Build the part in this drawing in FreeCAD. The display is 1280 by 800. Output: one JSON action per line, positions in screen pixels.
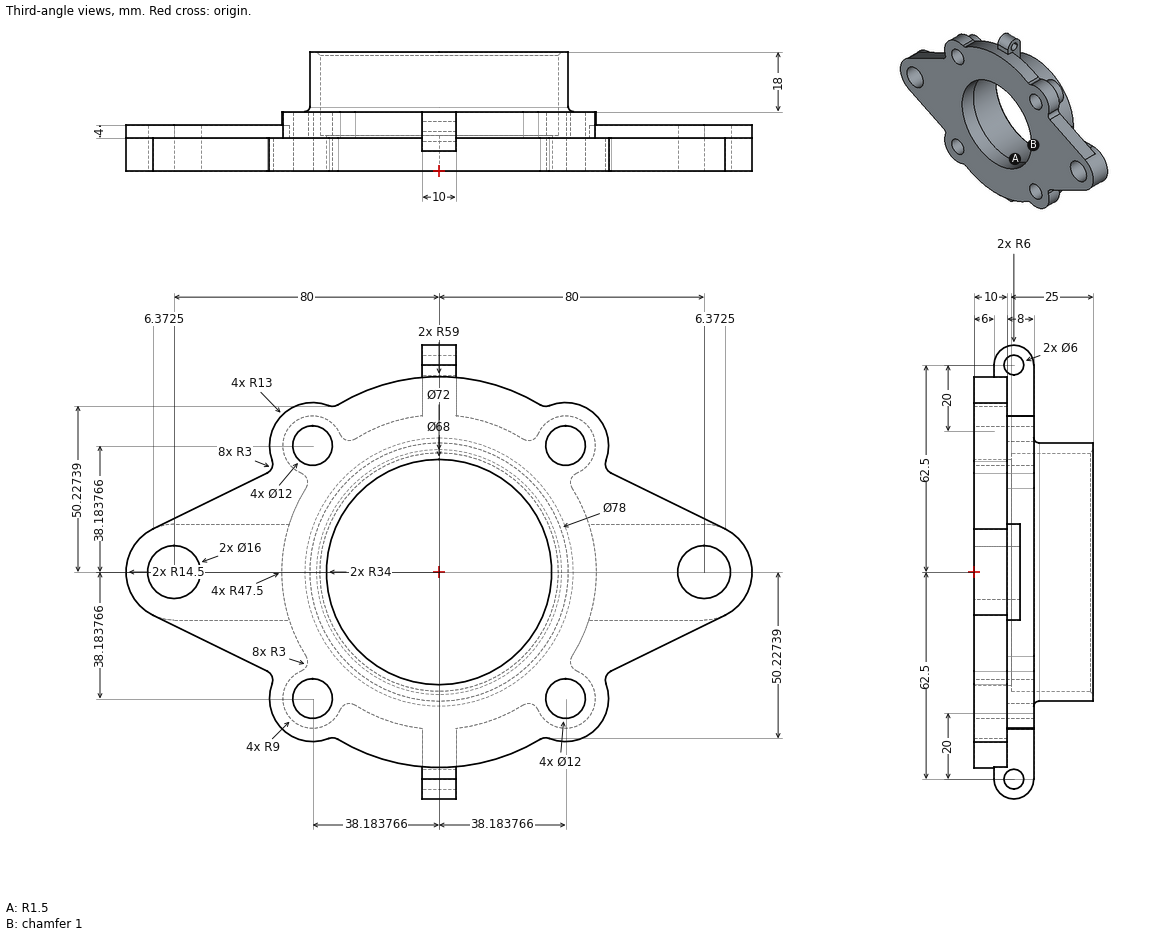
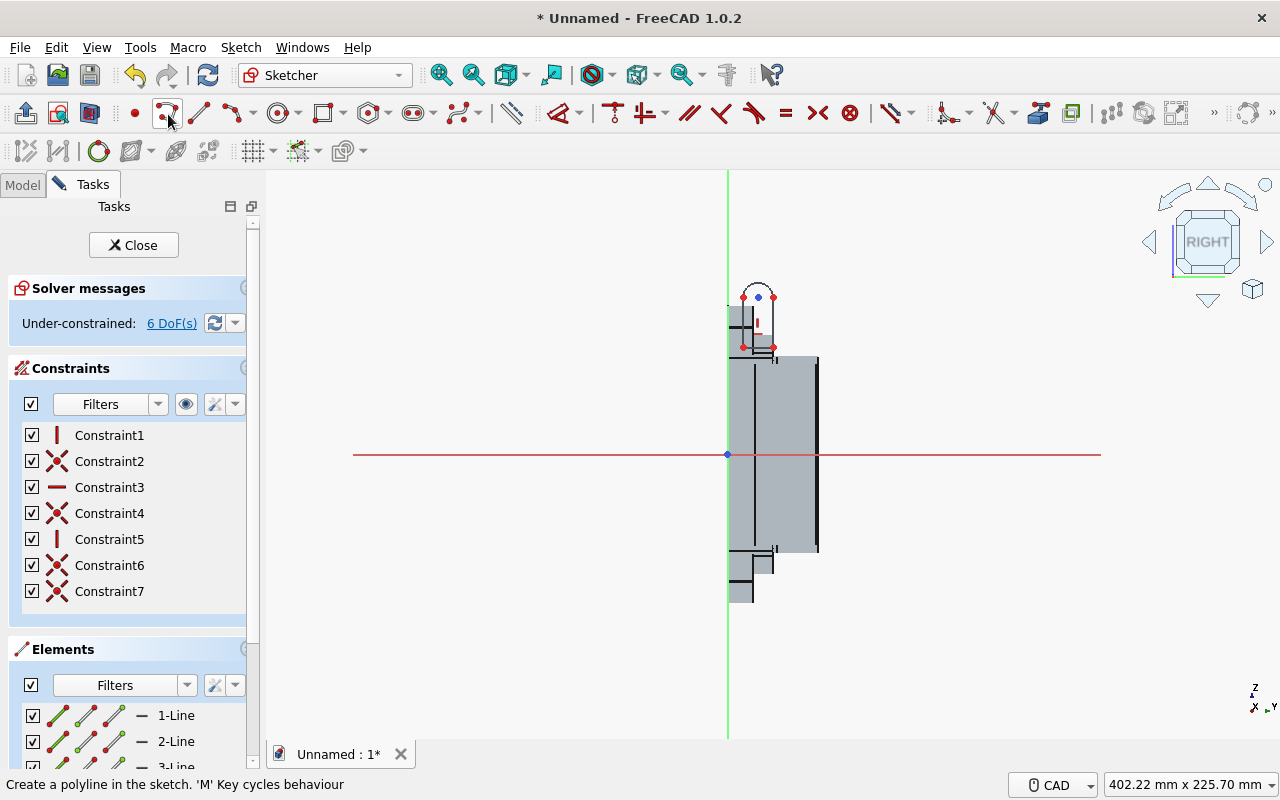
{"action": "left_click", "coordinate": [773, 612]}
{"action": "left_click", "coordinate": [773, 562]}
{"action": "left_click", "coordinate": [743, 562]}
{"action": "left_click", "coordinate": [743, 612]}
{"action": "right_click", "coordinate": [743, 612]}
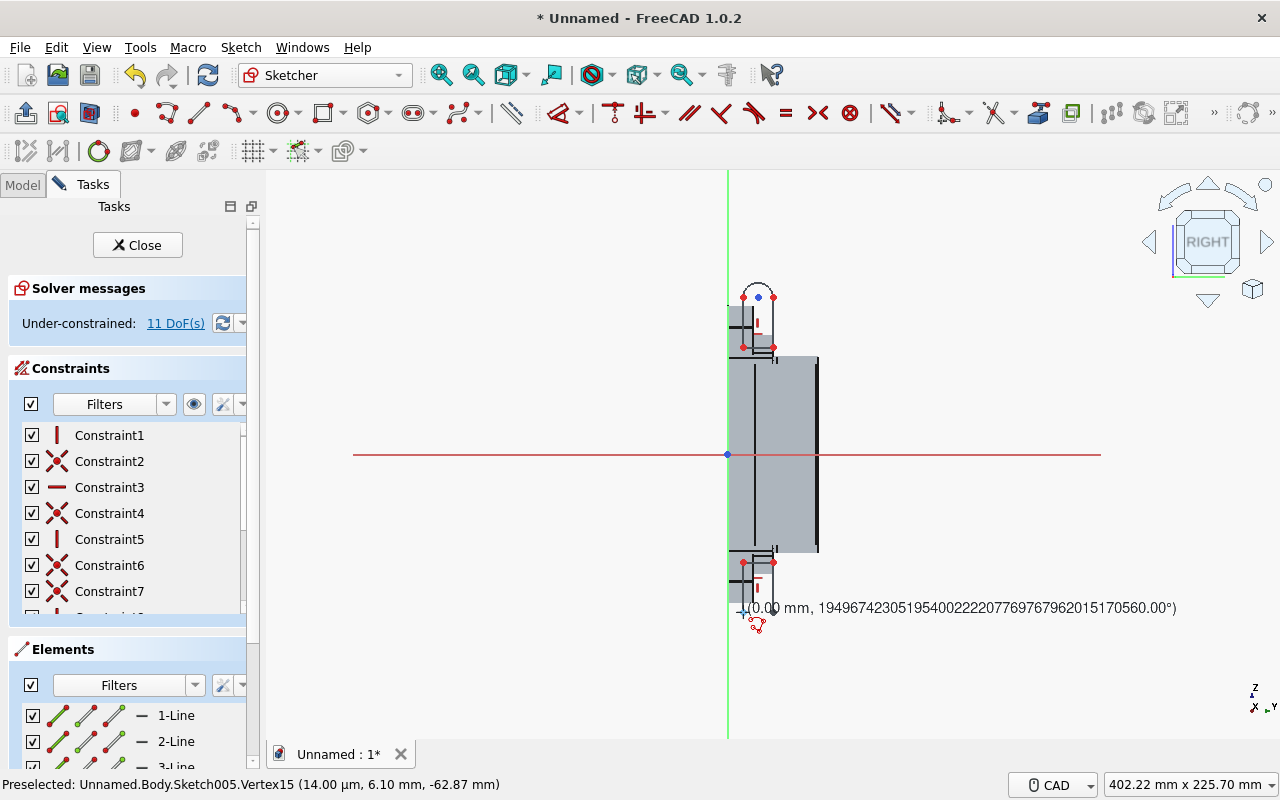
{"action": "left_click", "coordinate": [232, 114]}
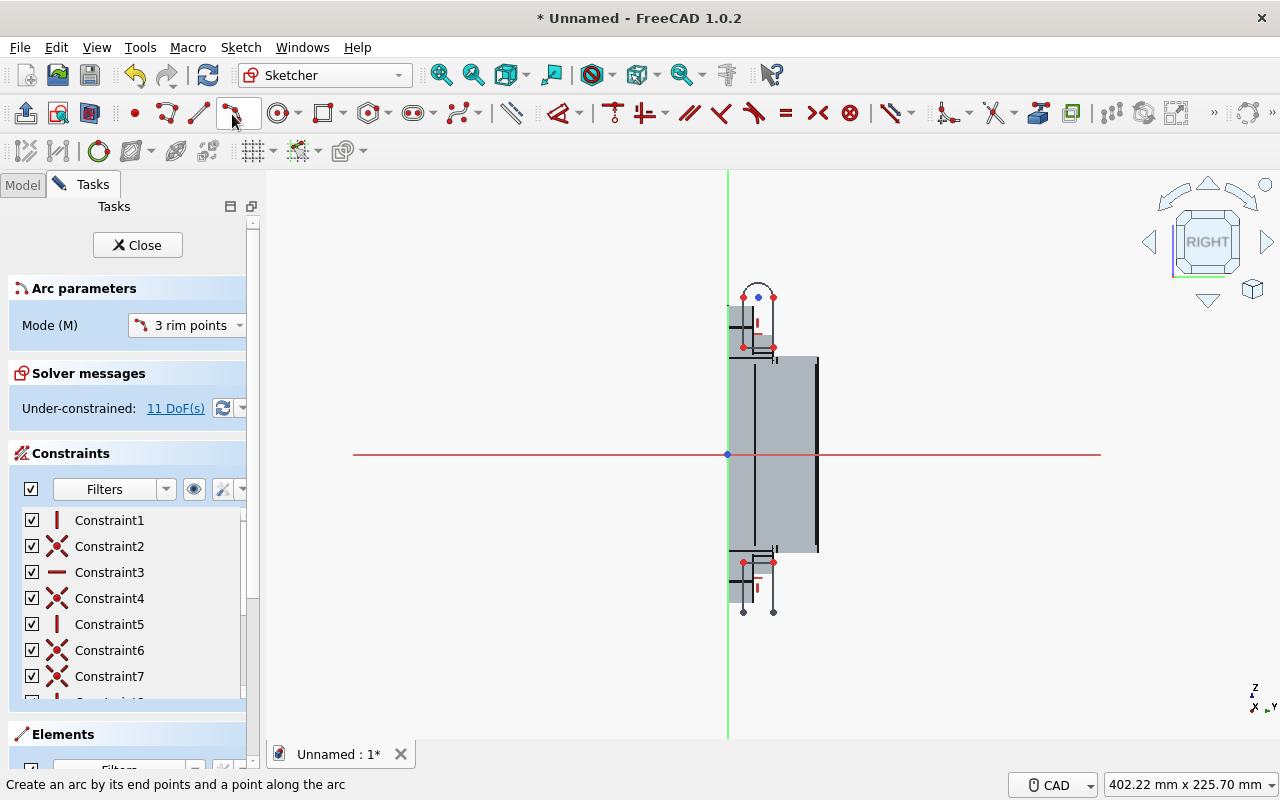
{"action": "left_click", "coordinate": [743, 613]}
{"action": "left_click", "coordinate": [773, 613]}
{"action": "left_click", "coordinate": [758, 627]}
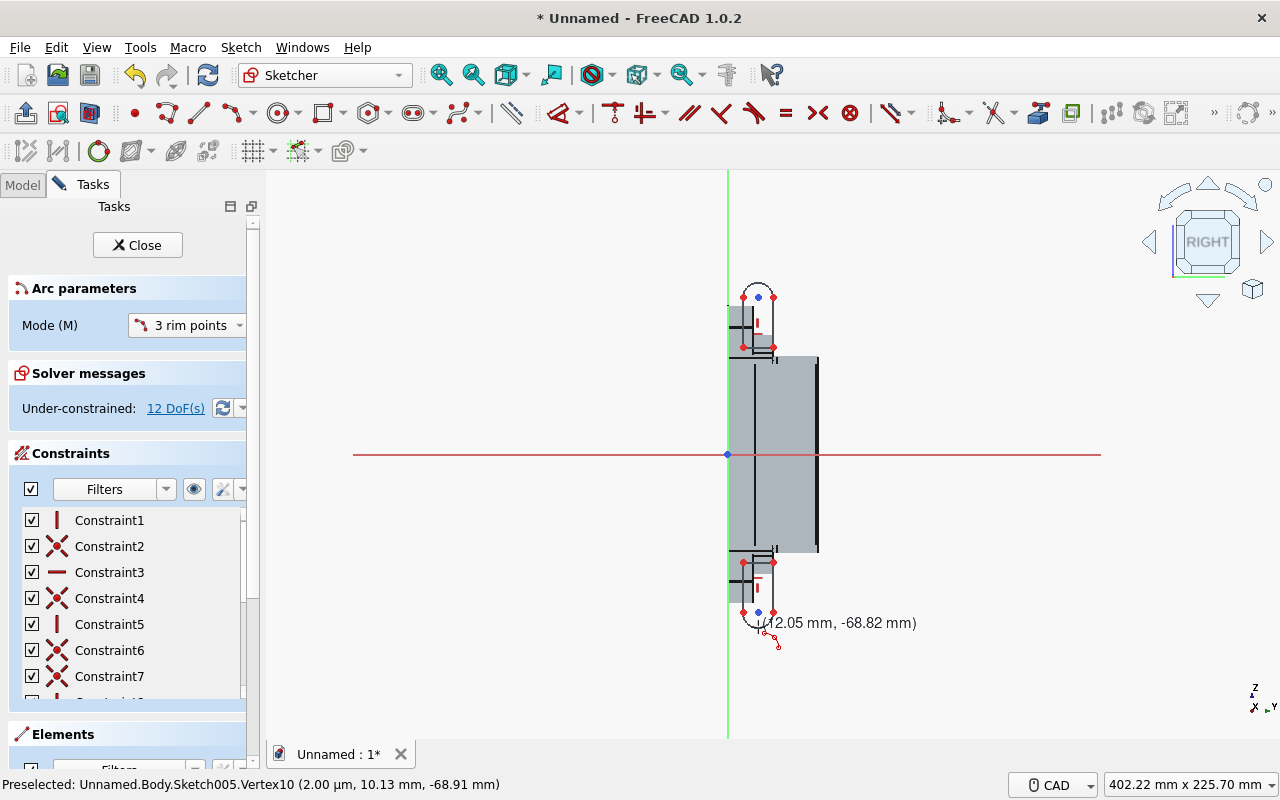
{"action": "left_click", "coordinate": [278, 114]}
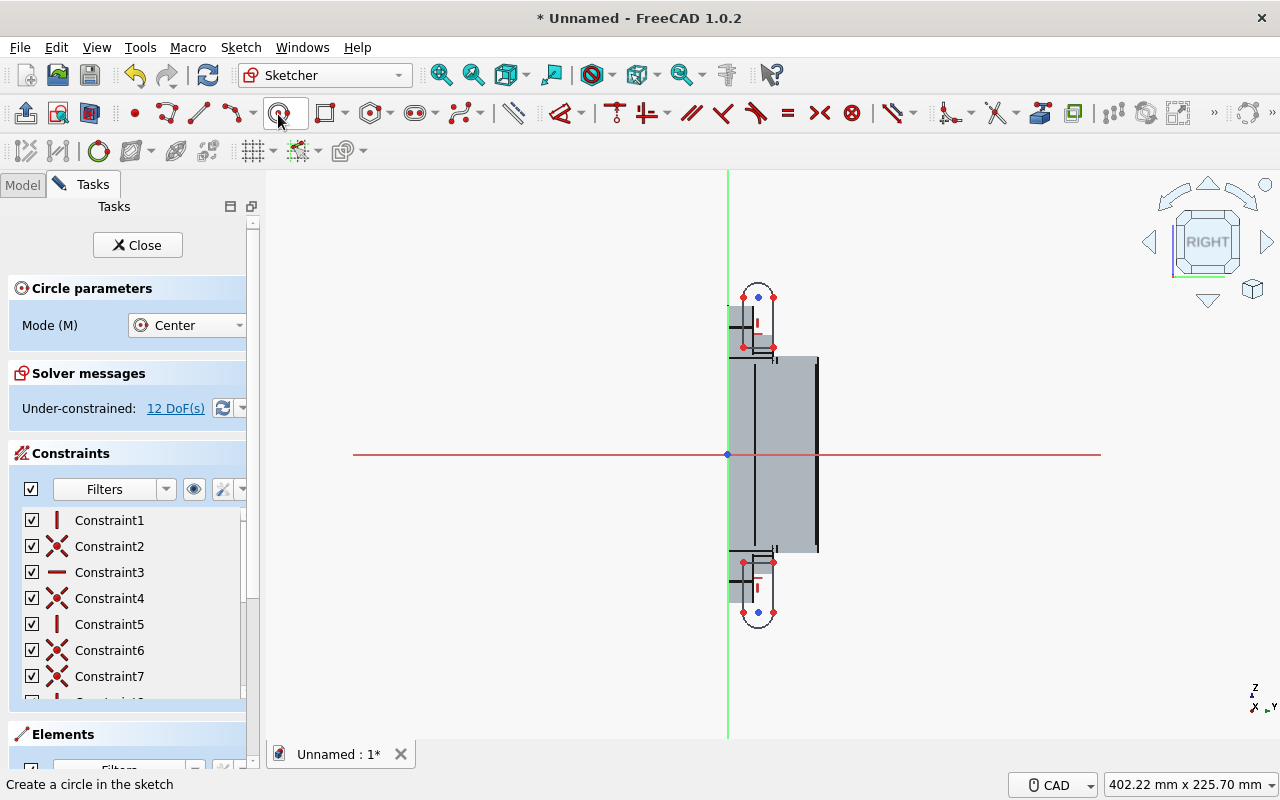
{"action": "scroll", "coordinate": [758, 297], "scroll_direction": "up", "scroll_amount": 6}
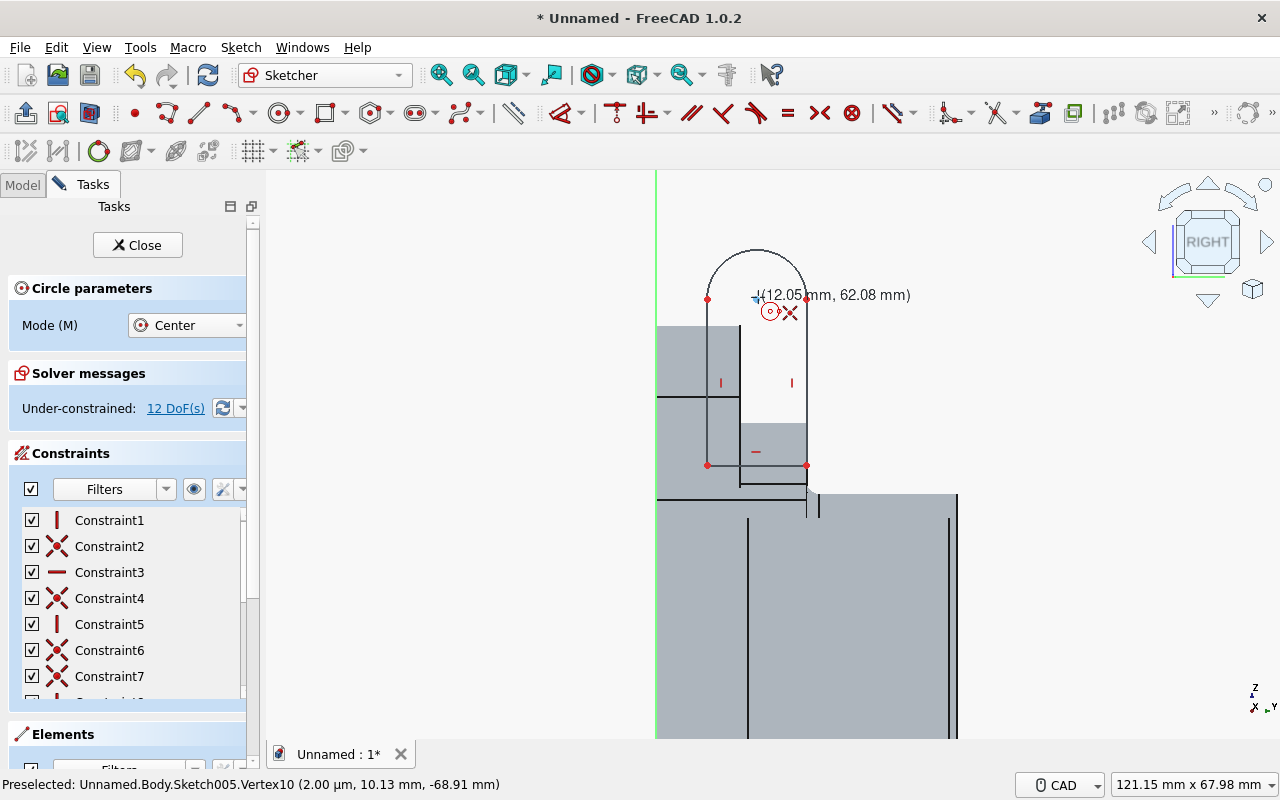
{"action": "left_click", "coordinate": [756, 296]}
{"action": "mouse_move", "coordinate": [774, 279]}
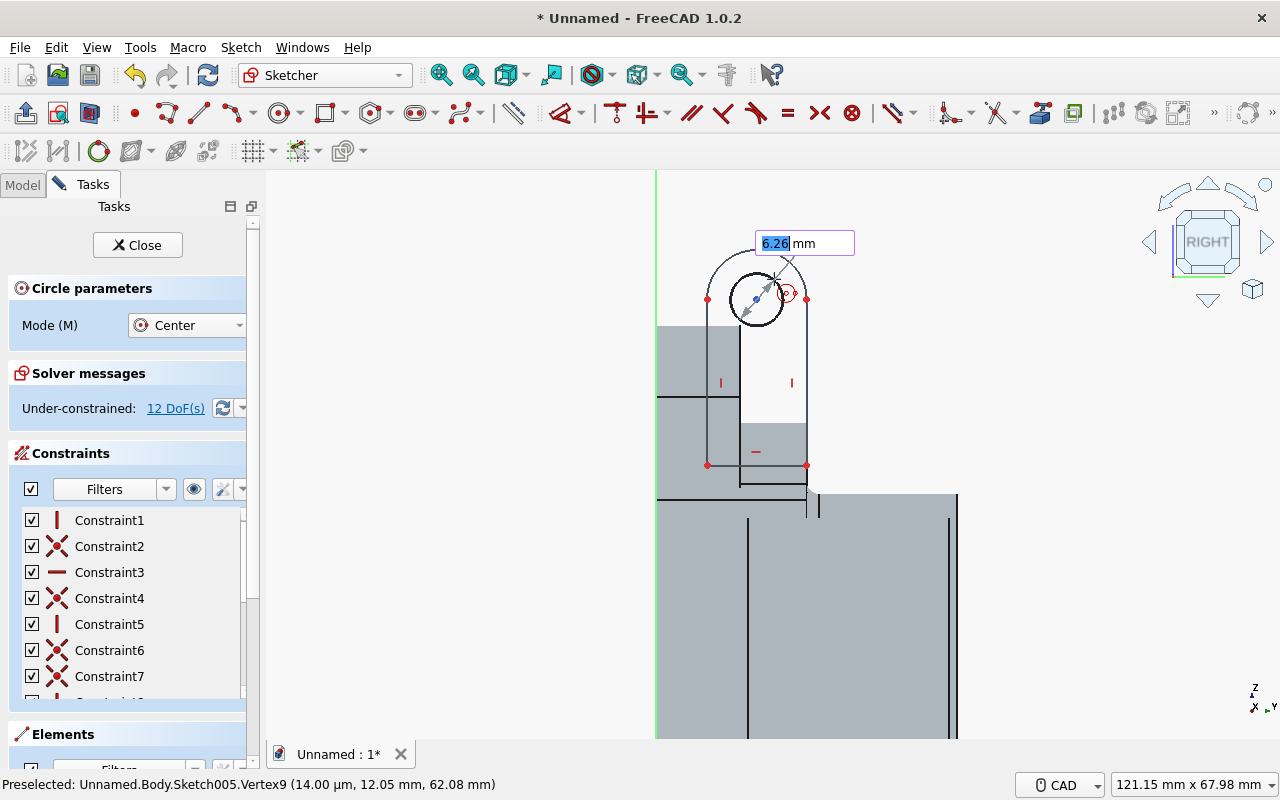
{"action": "type", "text": "6"}
{"action": "key", "text": "Return"}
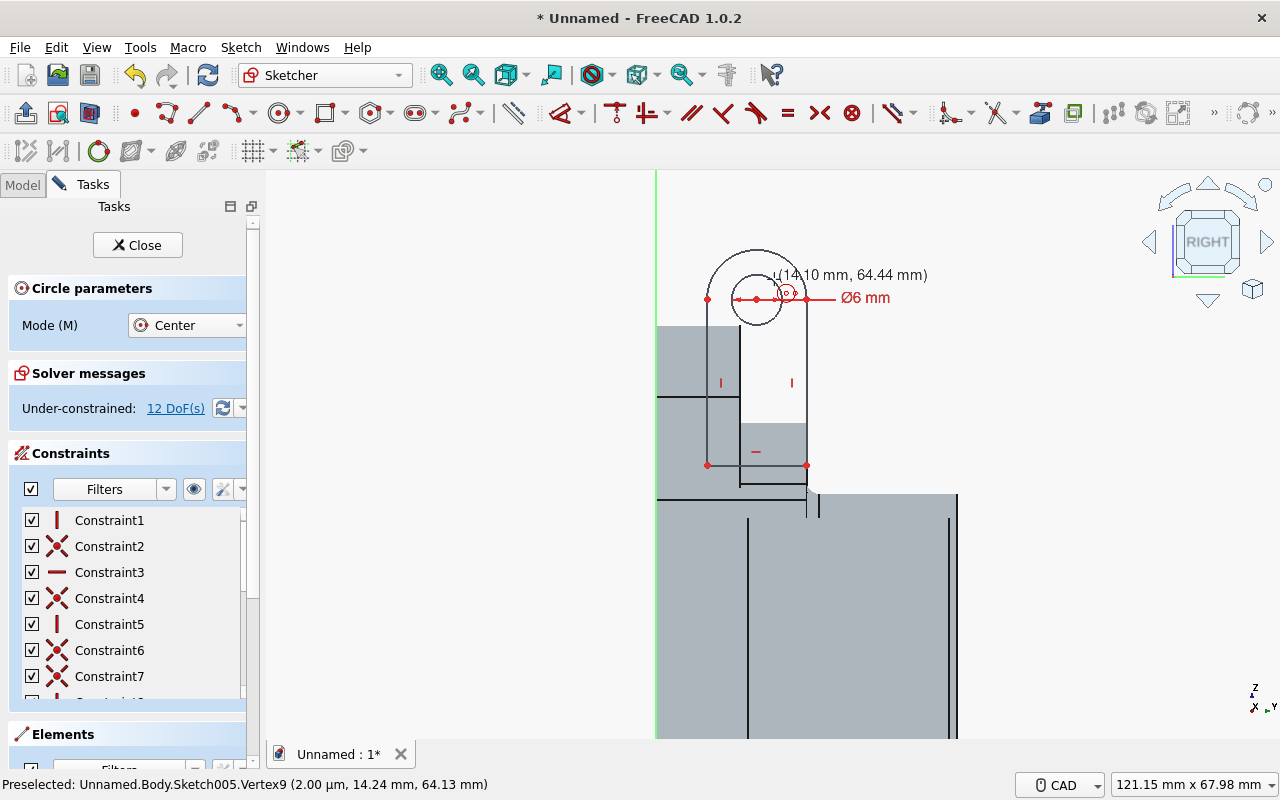
{"action": "scroll", "coordinate": [693, 297], "scroll_direction": "down", "scroll_amount": 6}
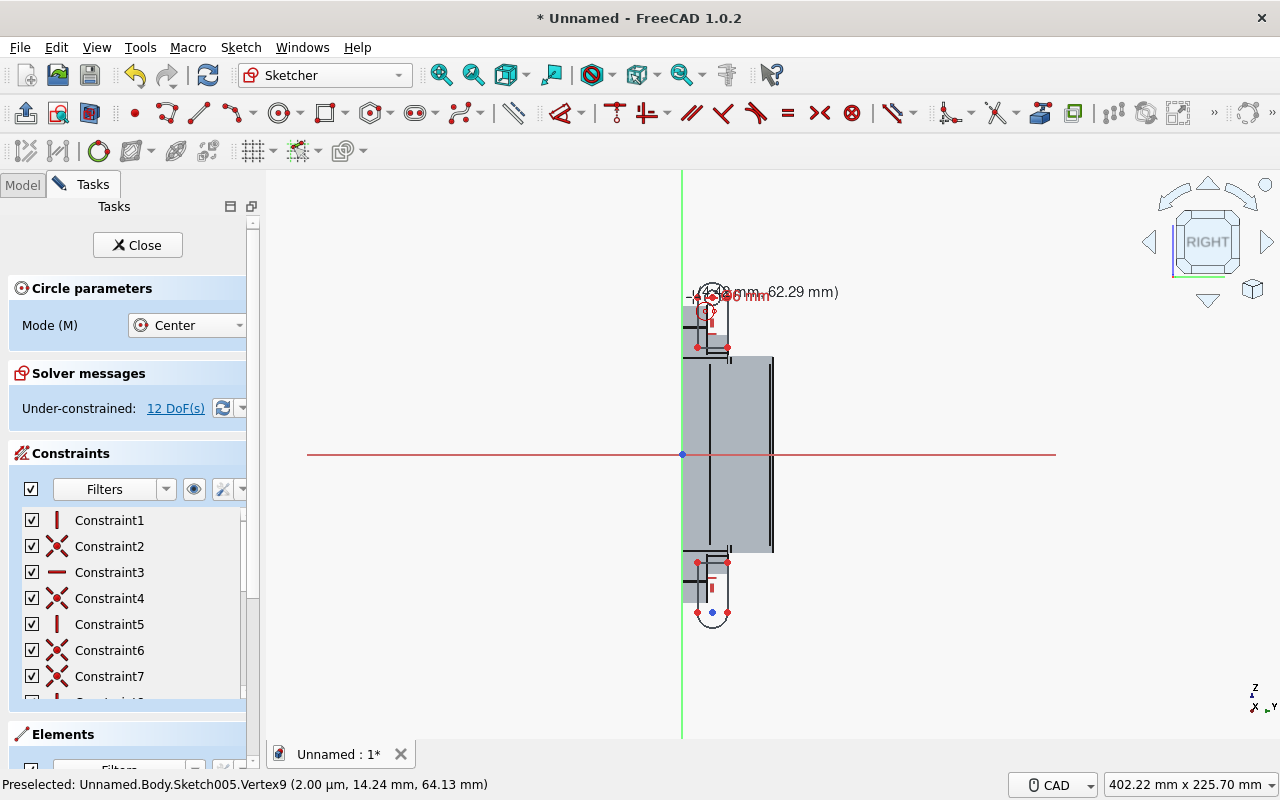
{"action": "scroll", "coordinate": [712, 612], "scroll_direction": "up", "scroll_amount": 6}